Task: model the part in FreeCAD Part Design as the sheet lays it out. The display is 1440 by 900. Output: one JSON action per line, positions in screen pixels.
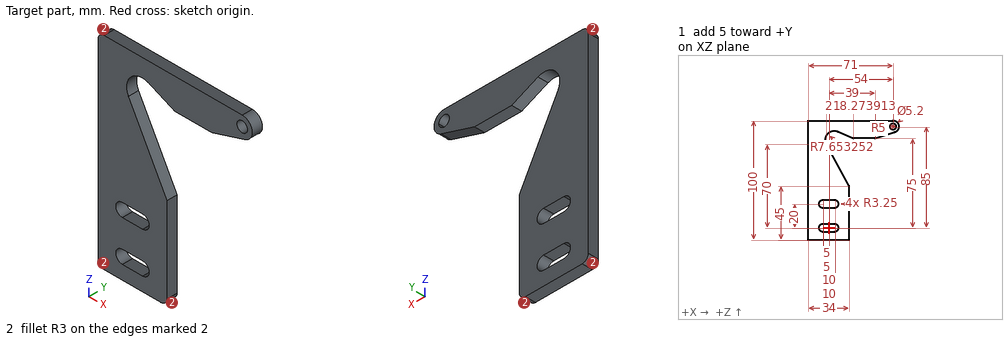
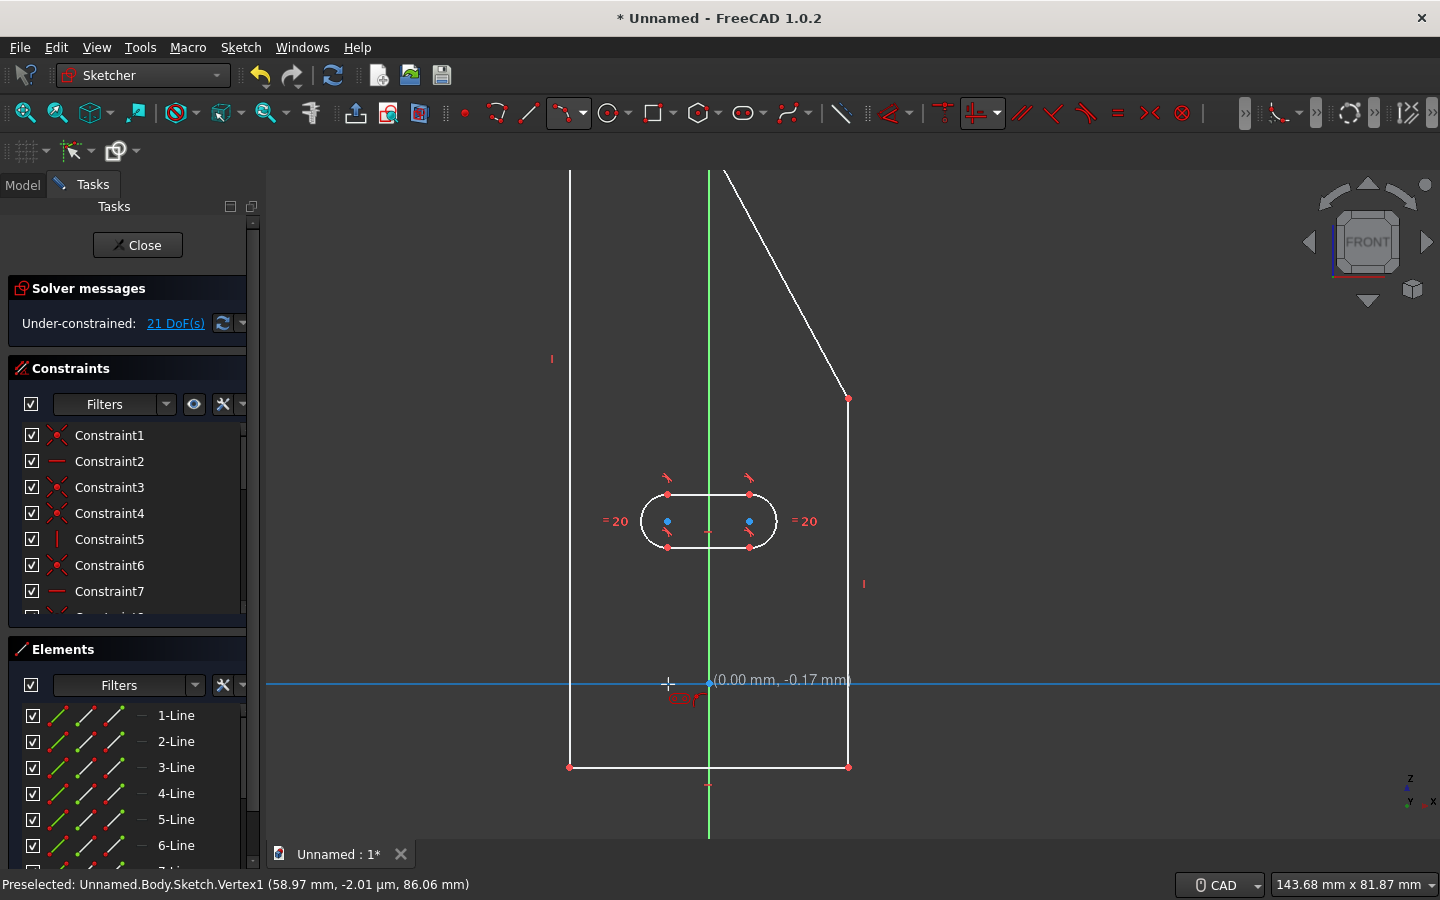
{"action": "left_click", "coordinate": [668, 684]}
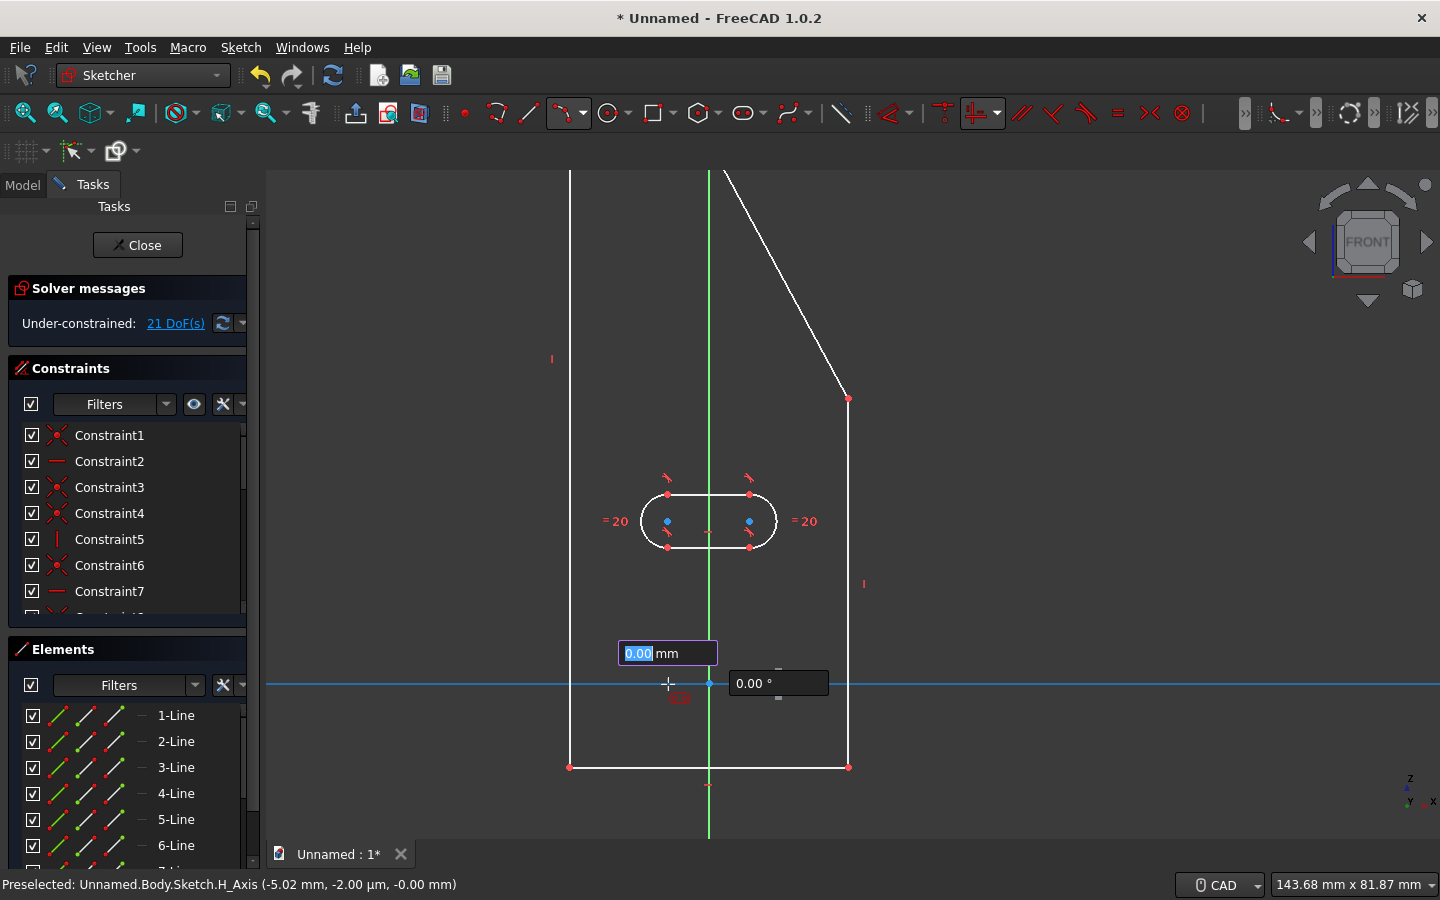
{"action": "left_click", "coordinate": [750, 675]}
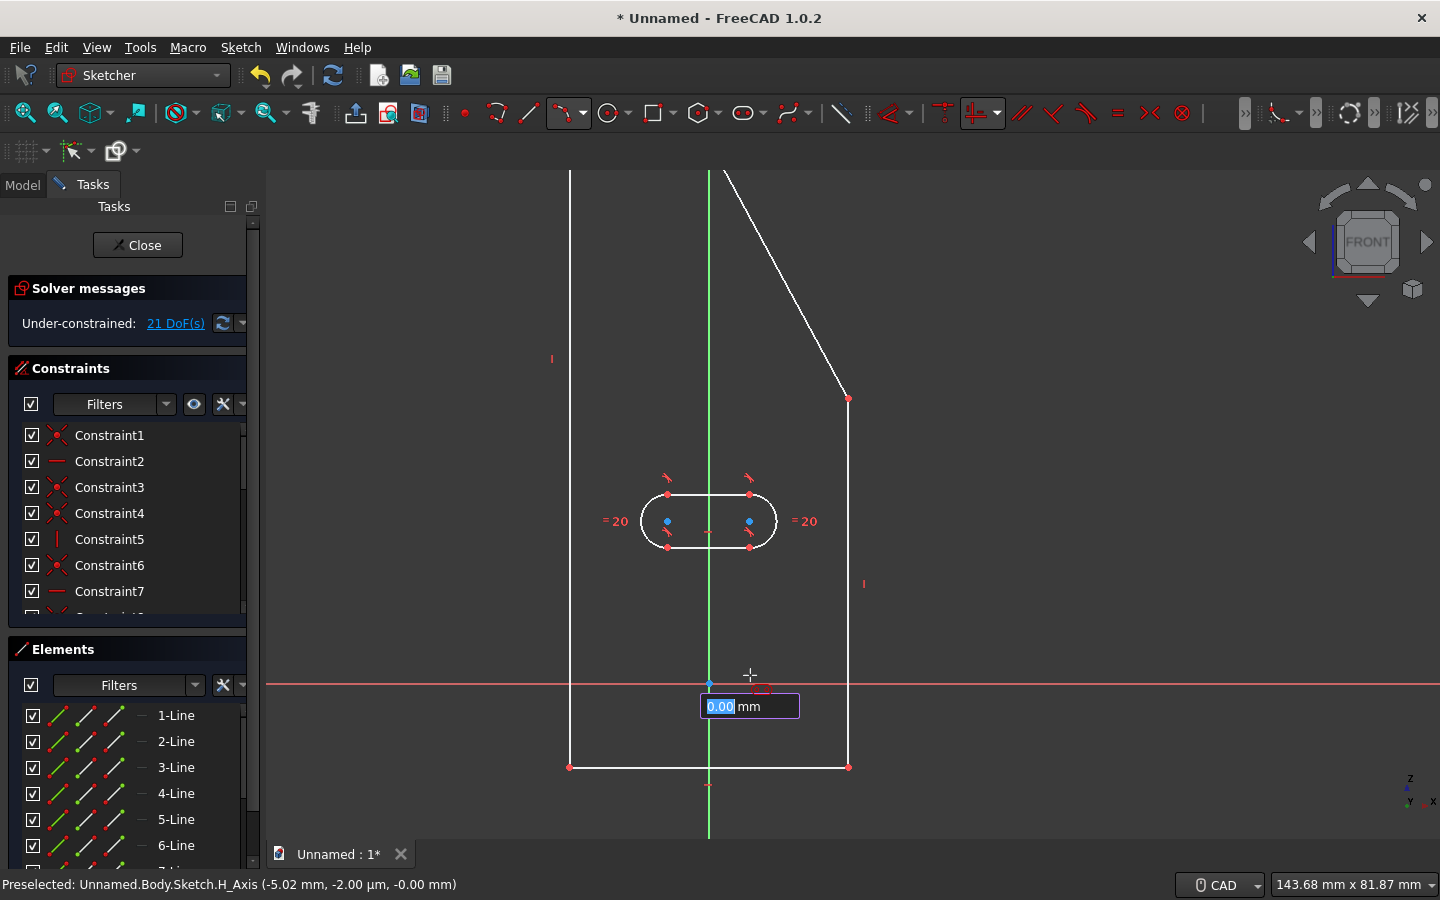
{"action": "scroll", "coordinate": [721, 657], "scroll_direction": "up", "scroll_amount": 2}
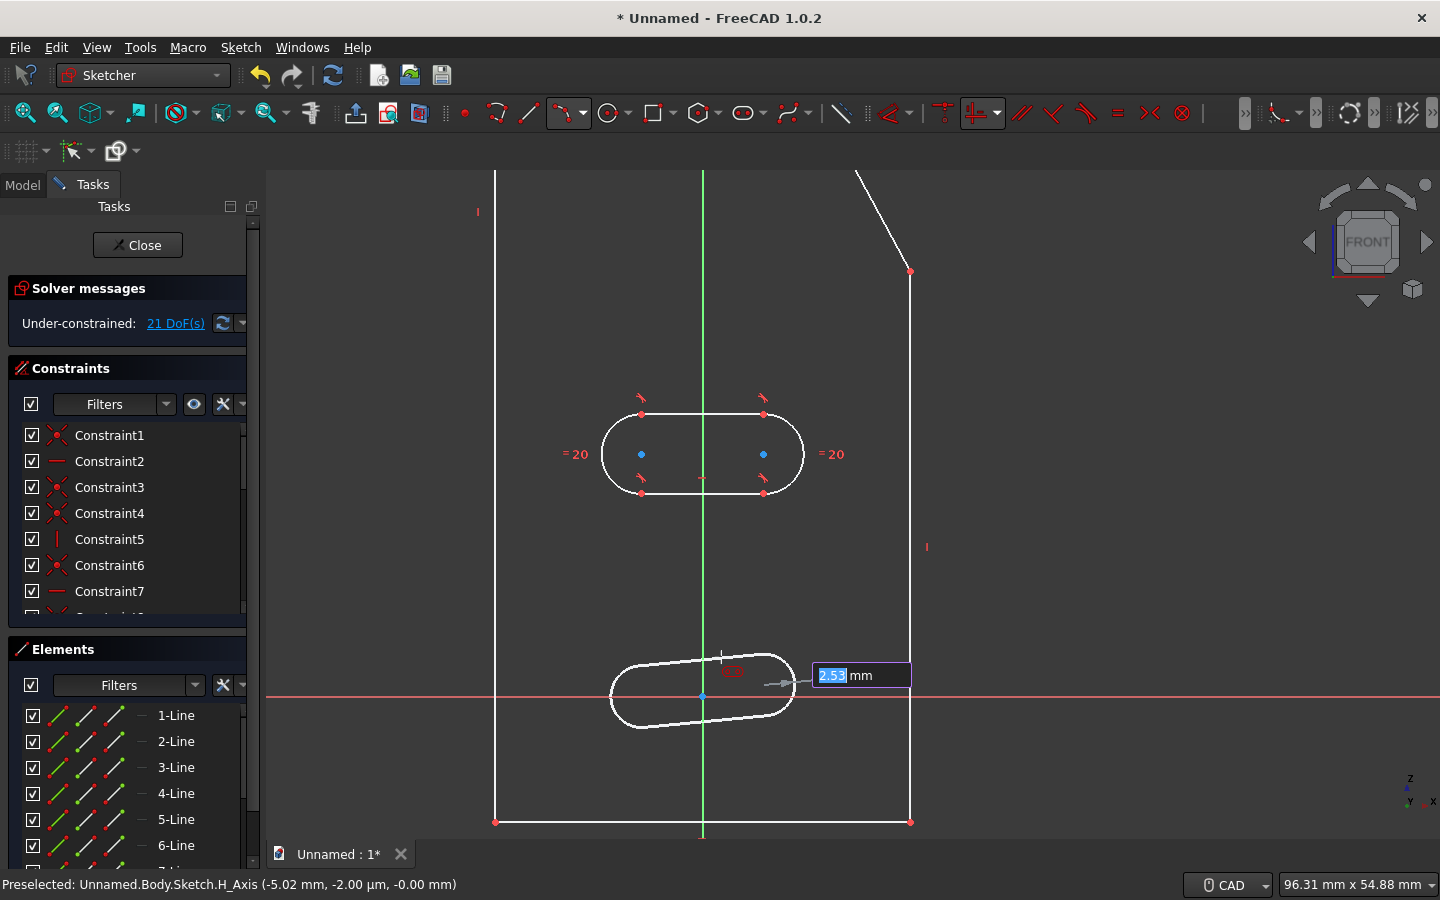
{"action": "left_click", "coordinate": [721, 657]}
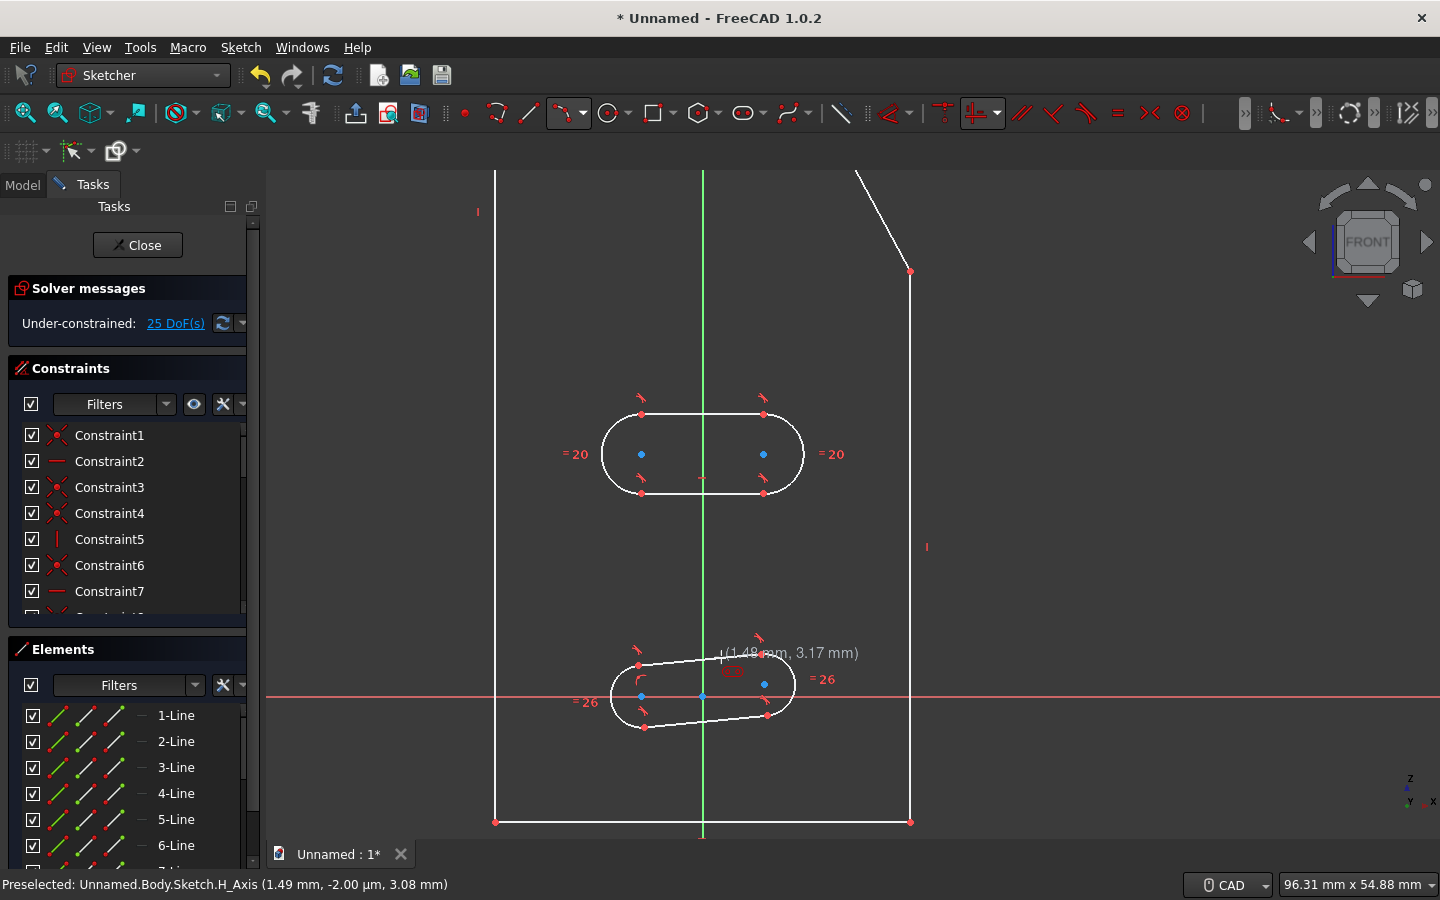
{"action": "left_click", "coordinate": [608, 114]}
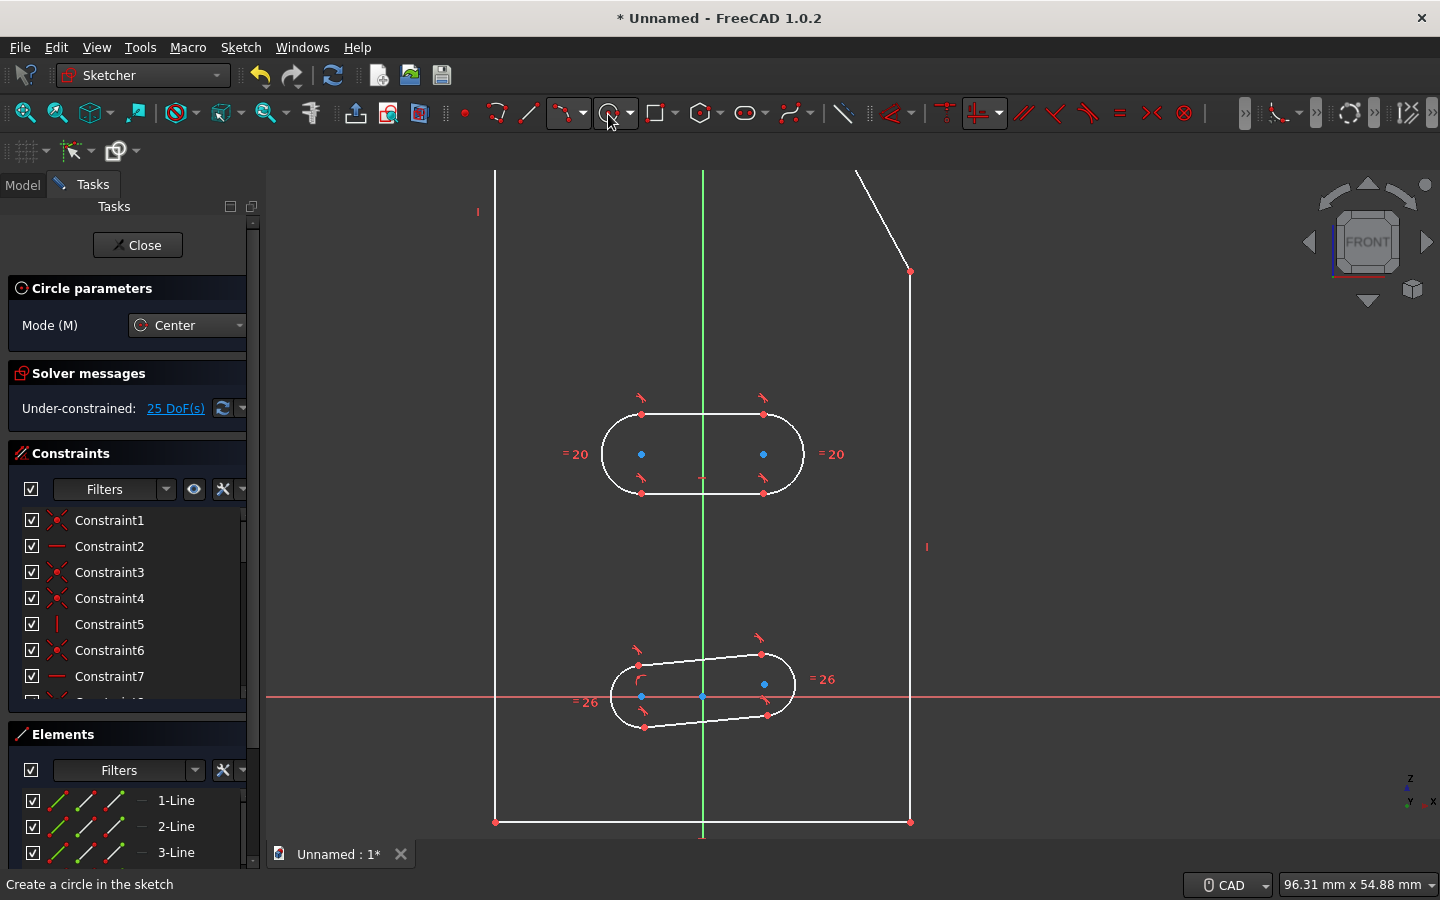
{"action": "scroll", "coordinate": [683, 676], "scroll_direction": "down", "scroll_amount": 5}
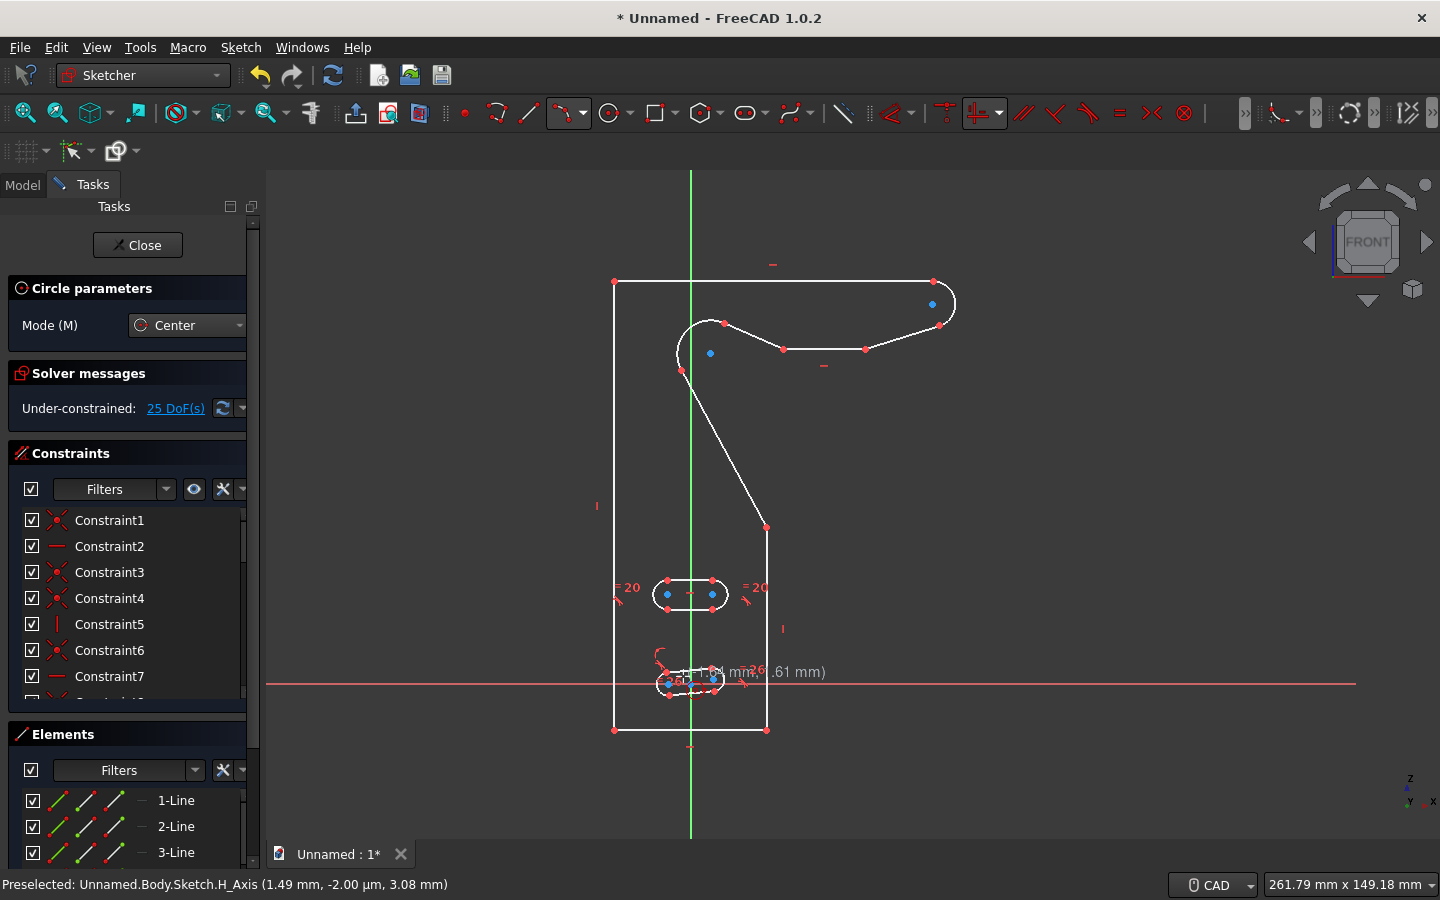
{"action": "scroll", "coordinate": [933, 303], "scroll_direction": "up", "scroll_amount": 4}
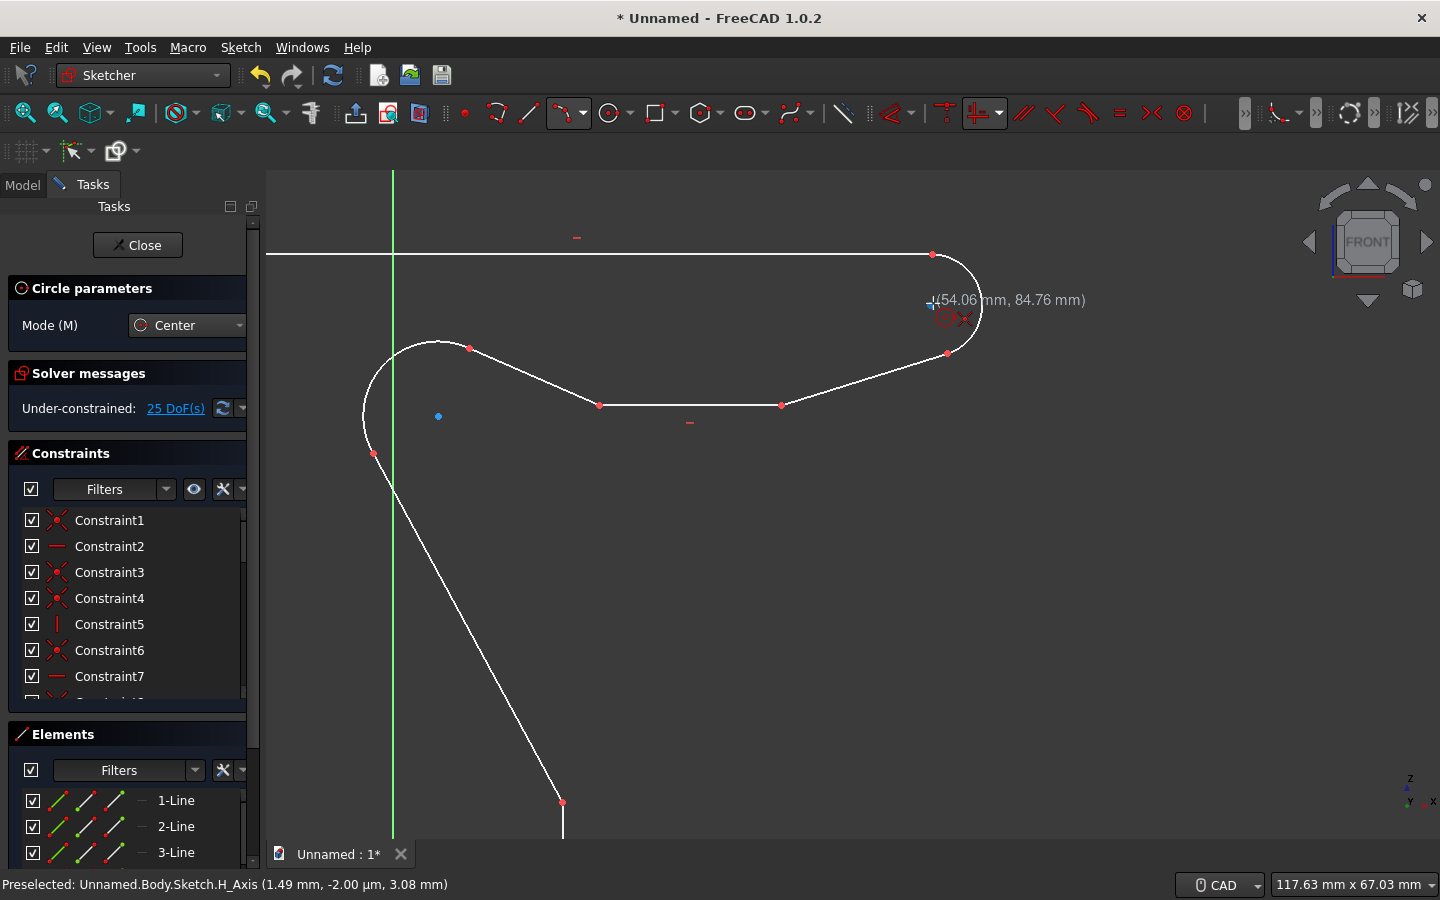
{"action": "left_click", "coordinate": [932, 303]}
{"action": "left_click", "coordinate": [950, 284]}
{"action": "key", "text": "Escape"}